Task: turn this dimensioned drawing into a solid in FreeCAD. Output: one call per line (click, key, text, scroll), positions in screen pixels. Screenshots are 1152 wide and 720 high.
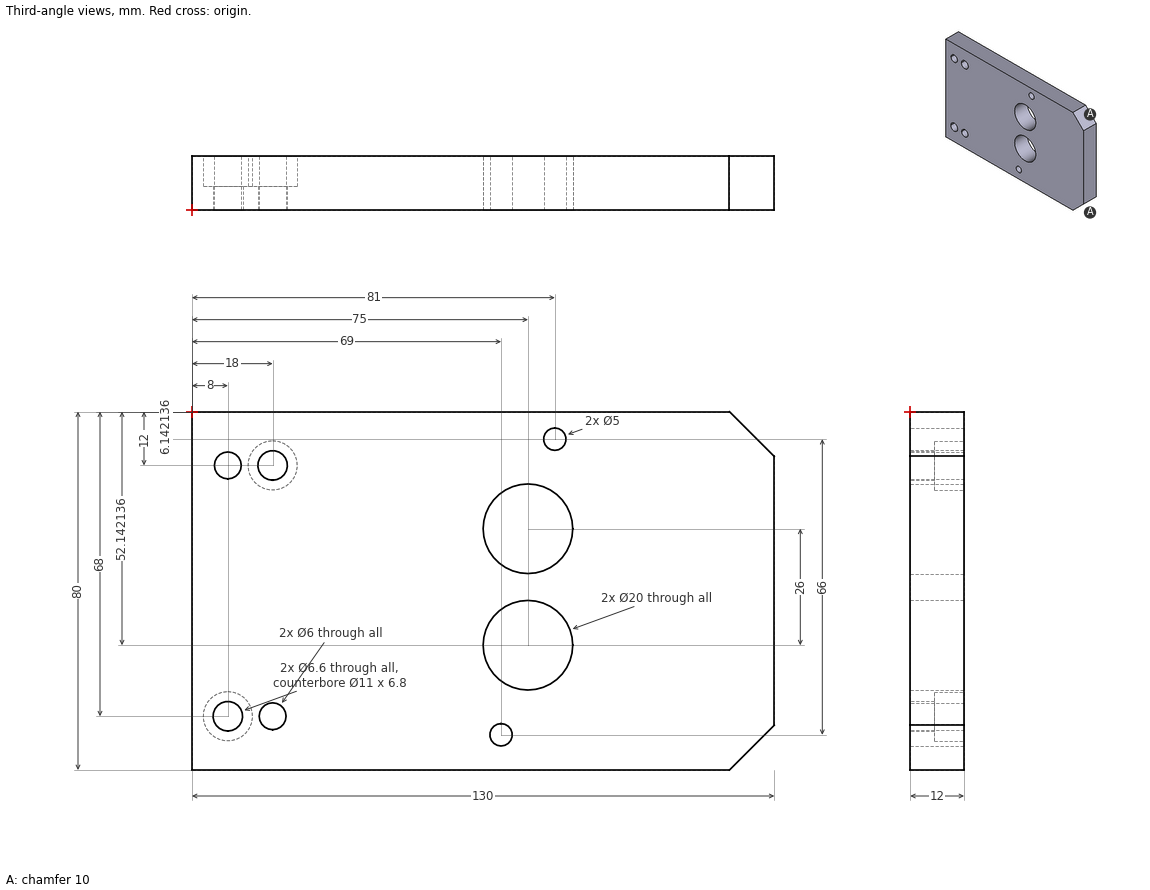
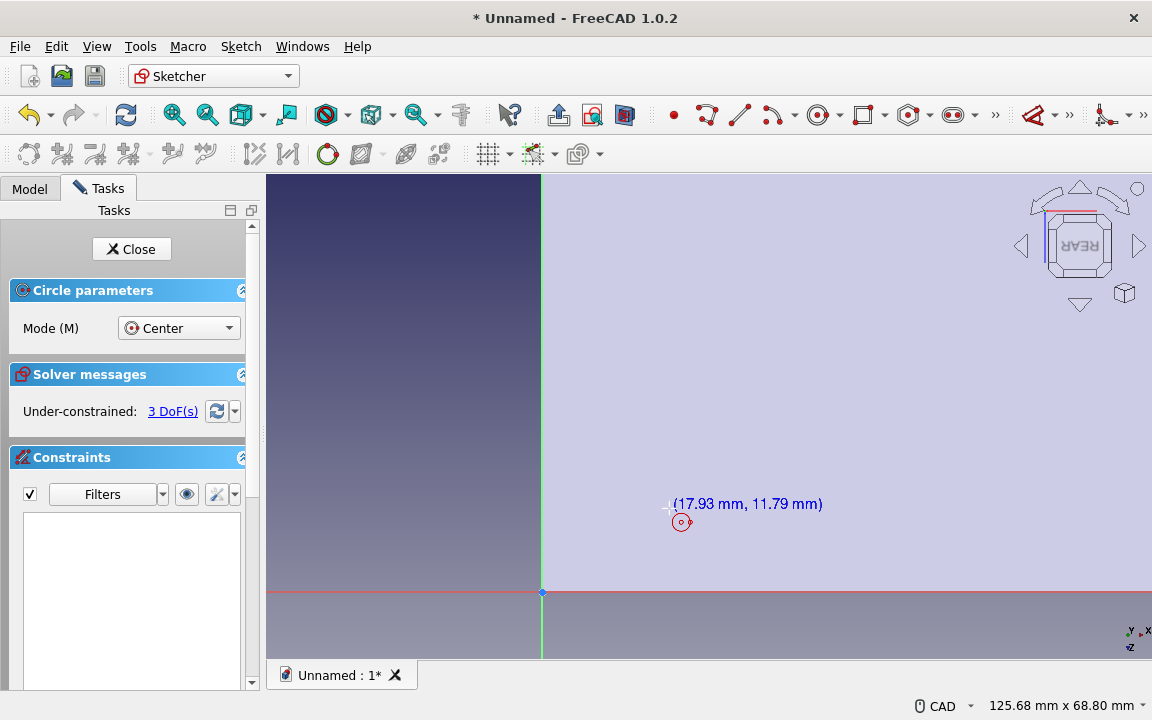
click(669, 508)
click(686, 491)
key(Escape)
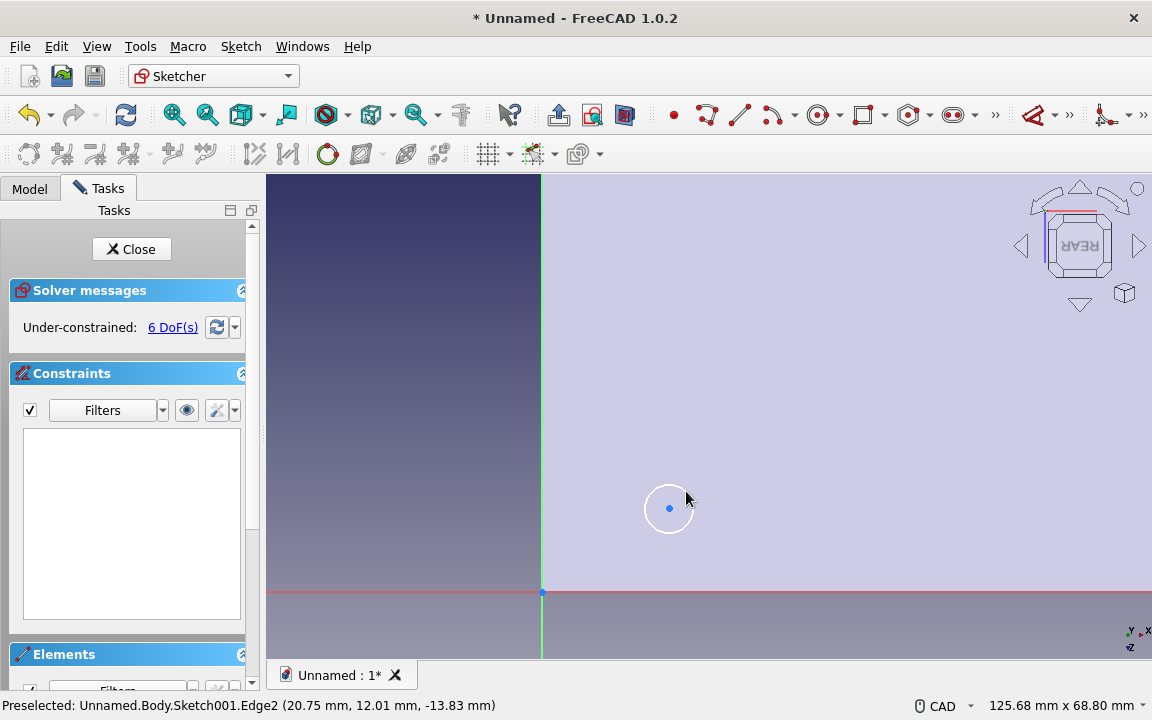
scroll(669, 508, down, 3)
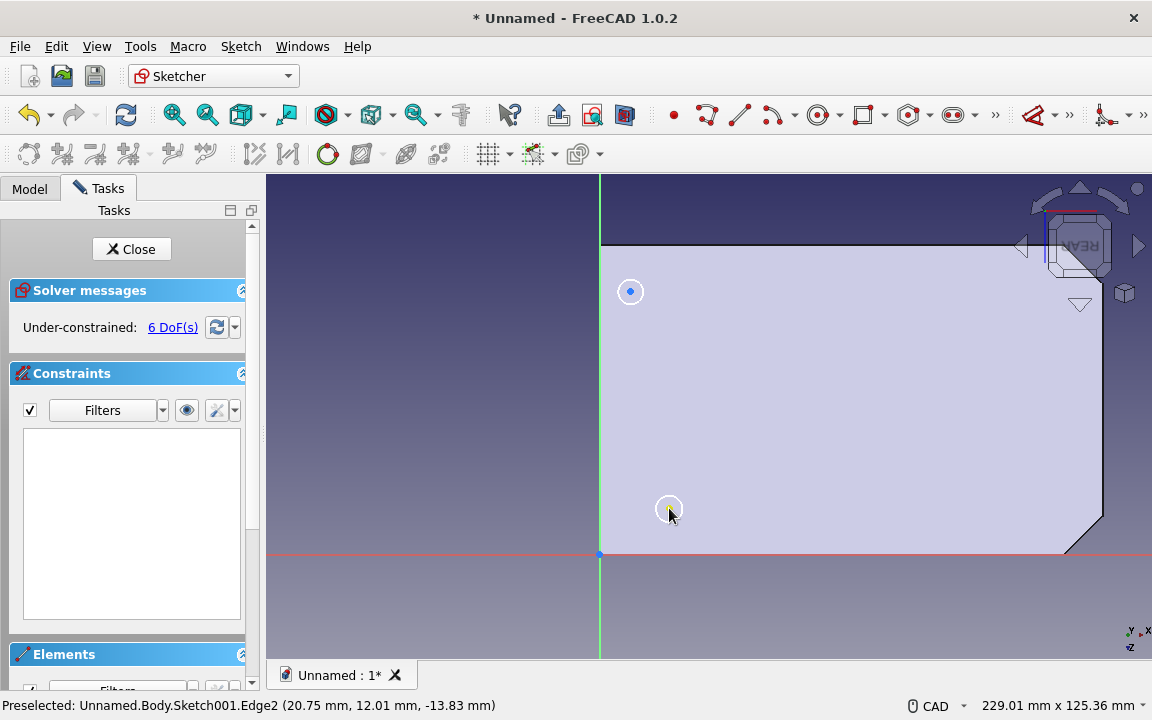
click(640, 283)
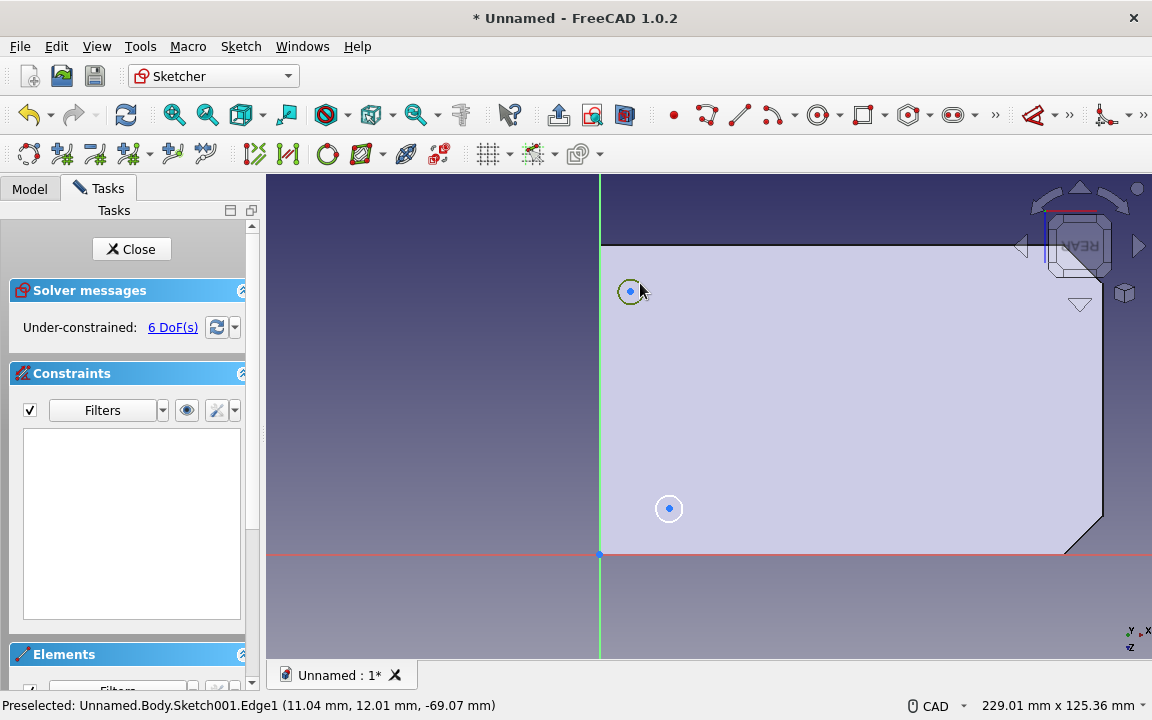
click(679, 500)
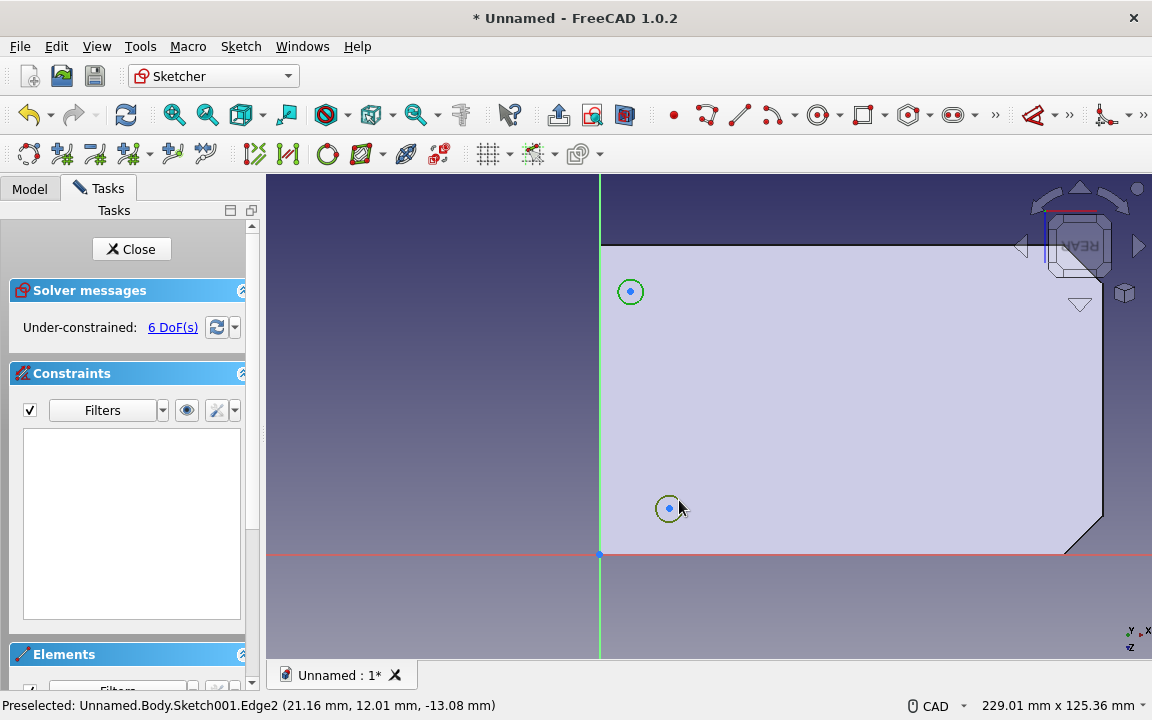
key(e)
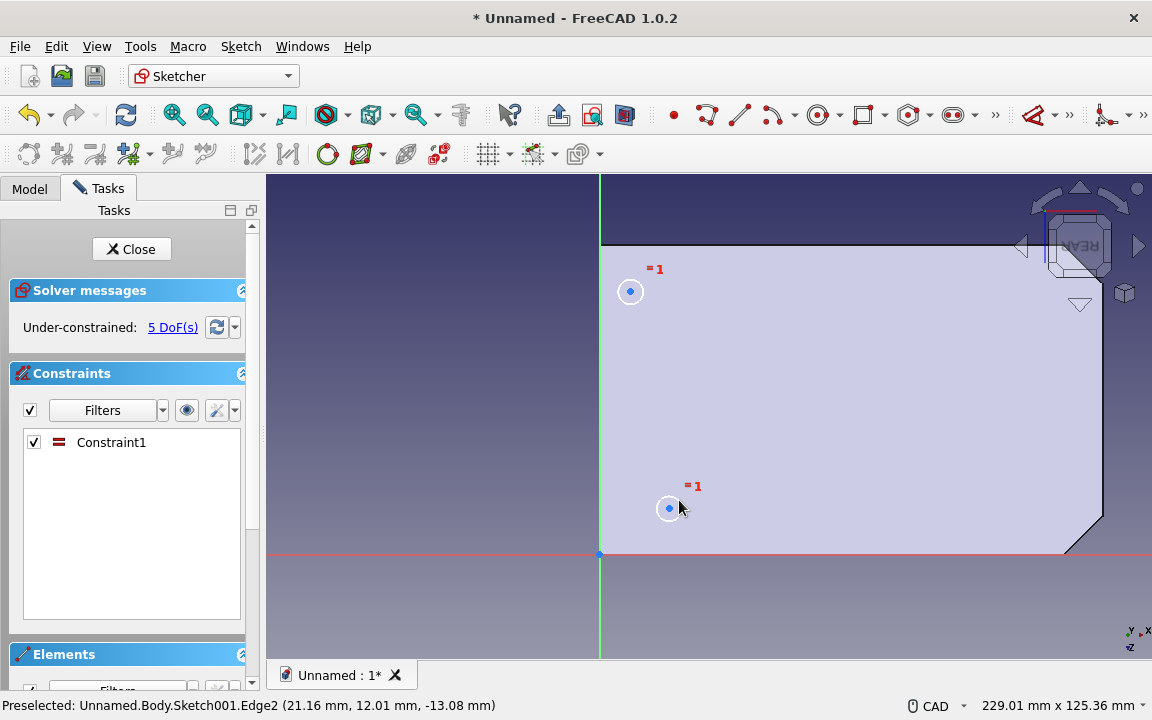
key(d)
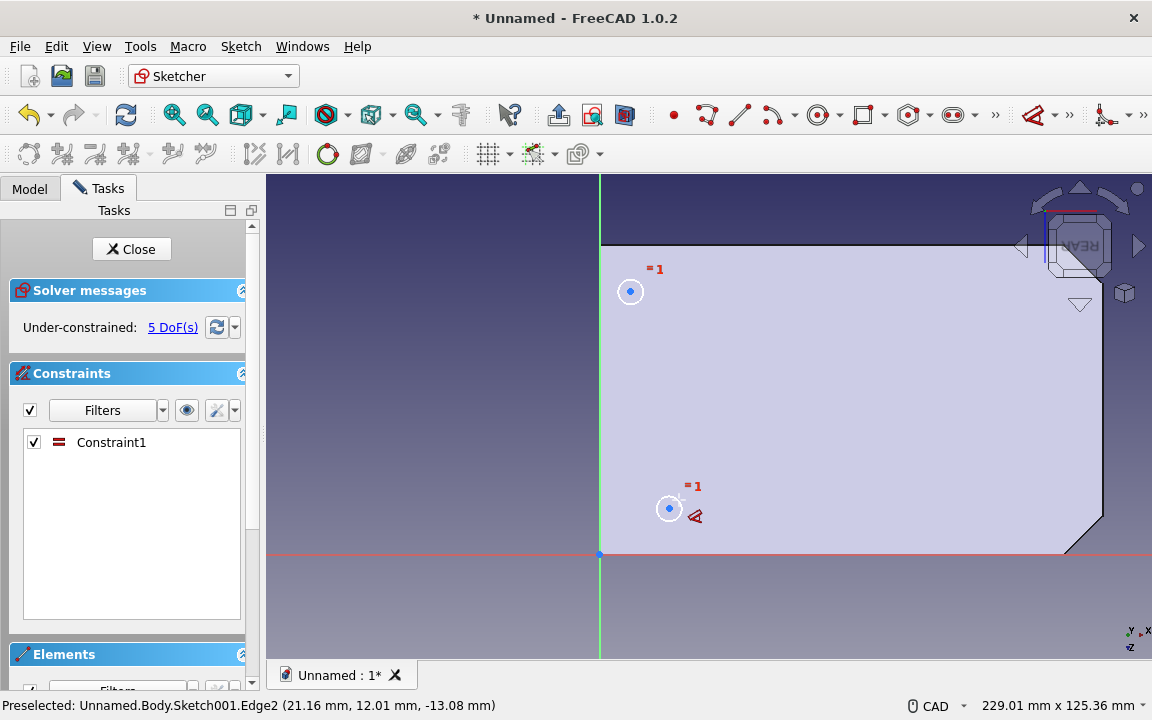
scroll(640, 283, up, 3)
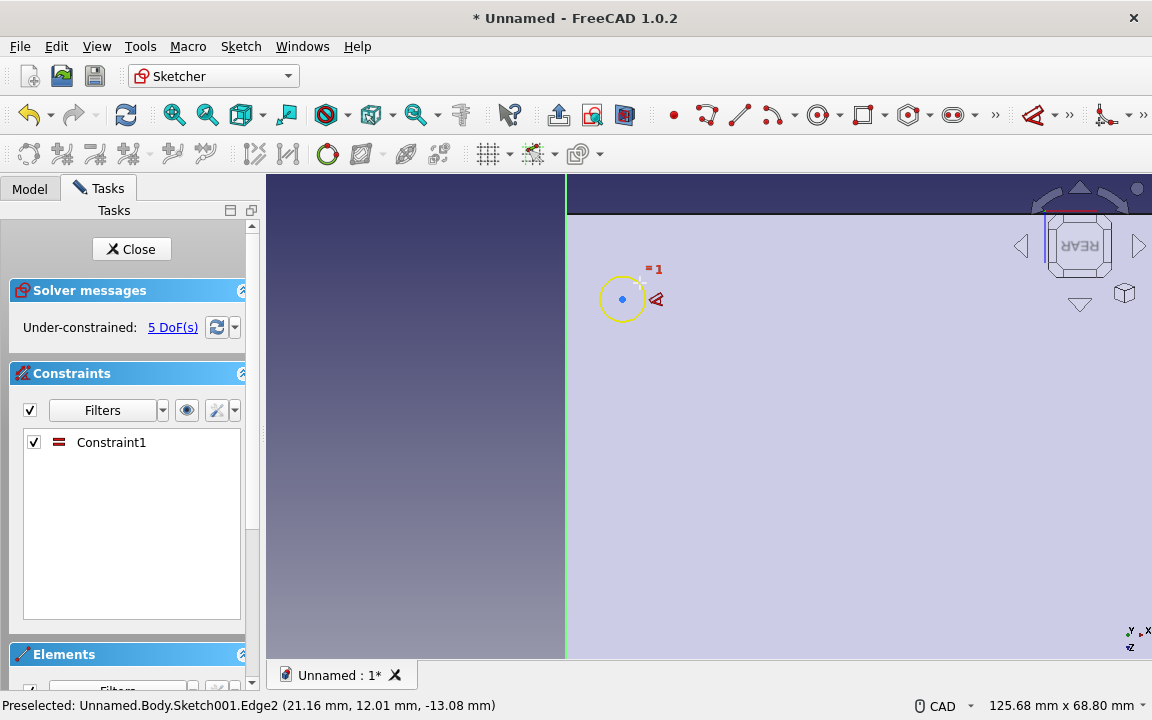
click(639, 283)
click(662, 260)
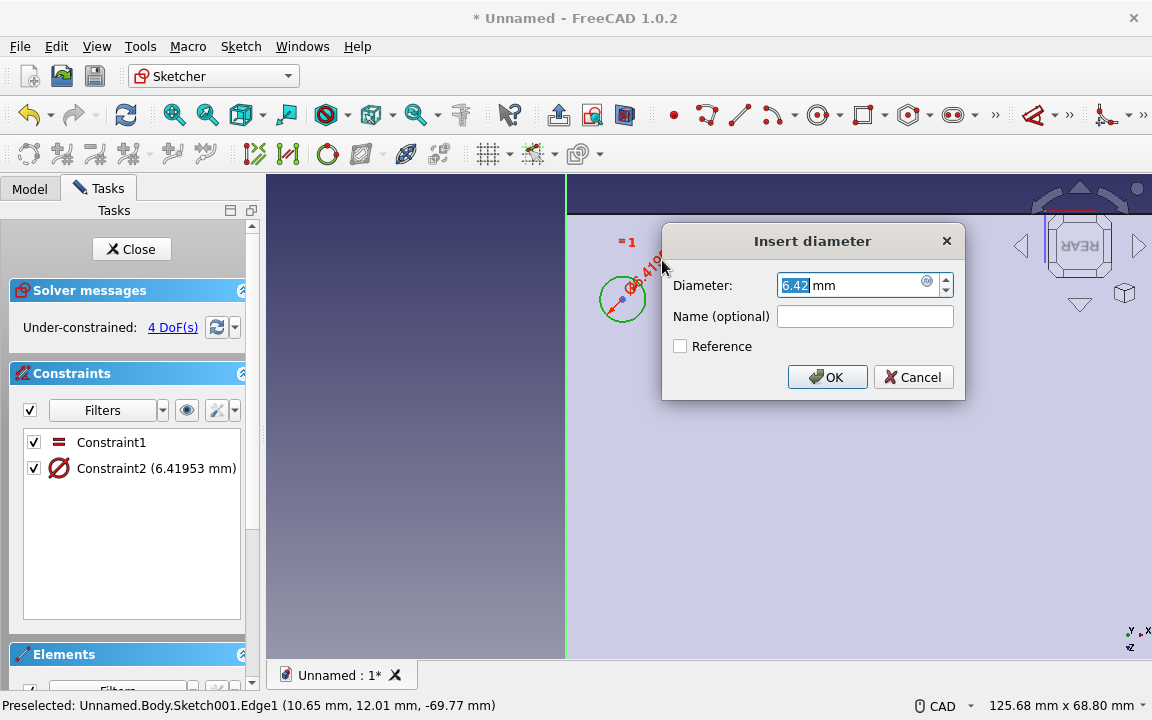
text(6.6)
key(Return)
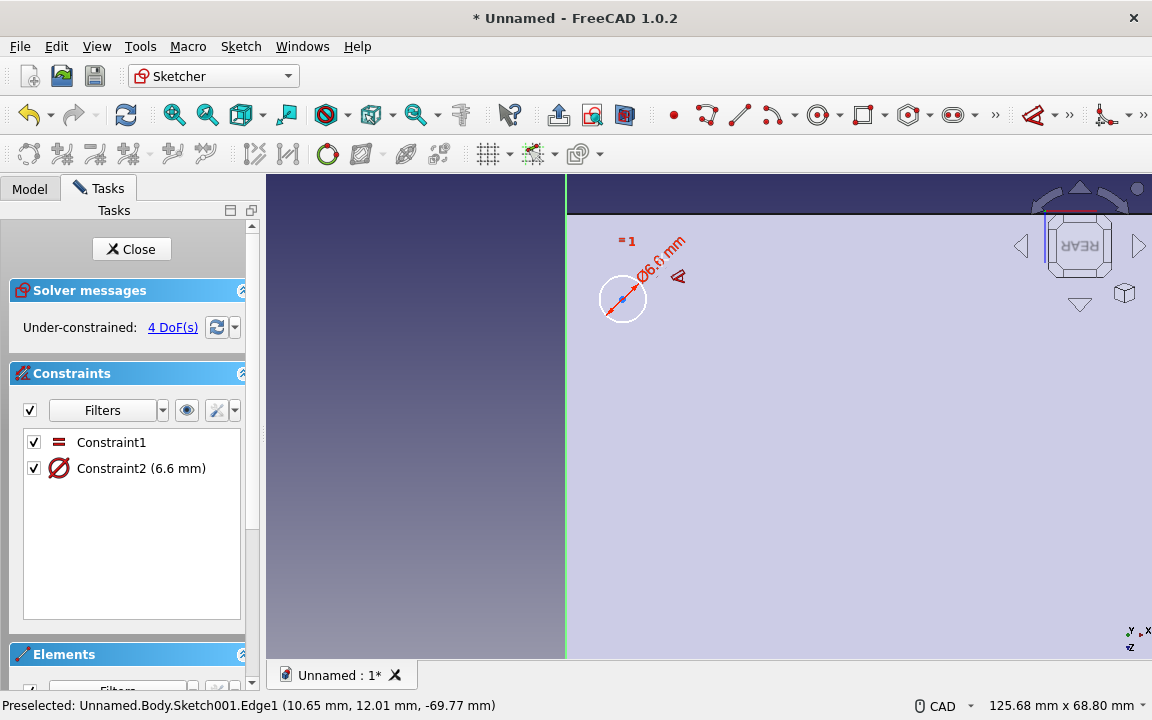
click(623, 299)
click(581, 265)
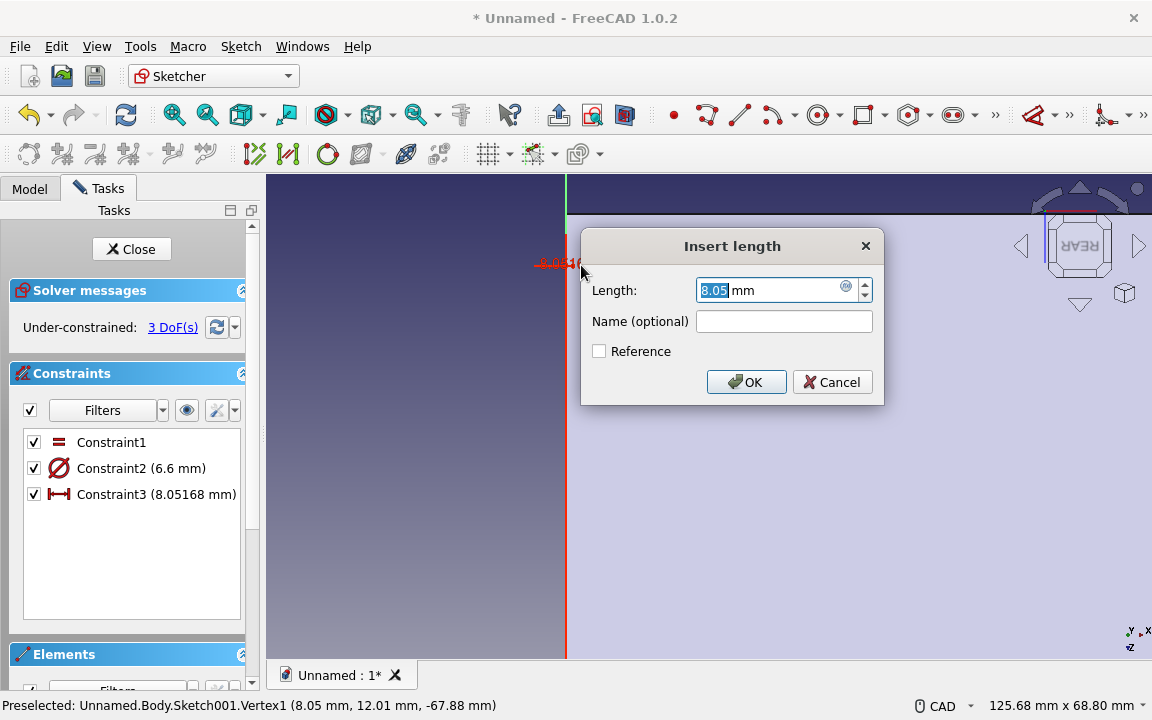
text(8)
key(Return)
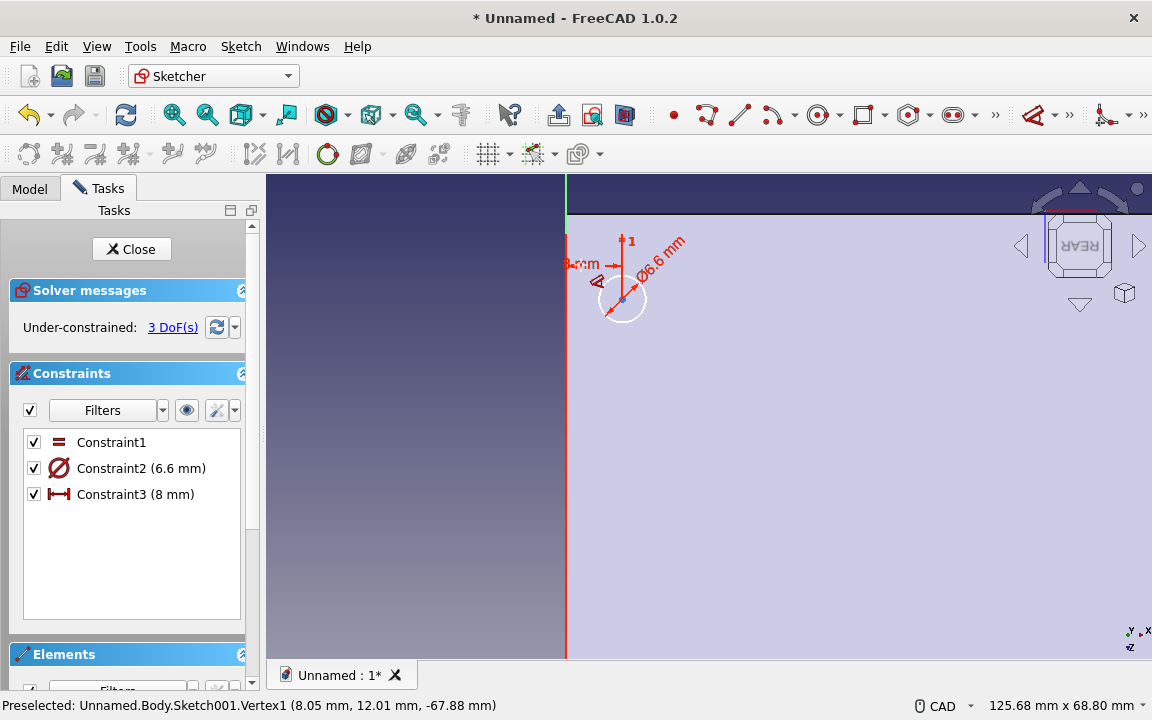
click(622, 299)
click(532, 465)